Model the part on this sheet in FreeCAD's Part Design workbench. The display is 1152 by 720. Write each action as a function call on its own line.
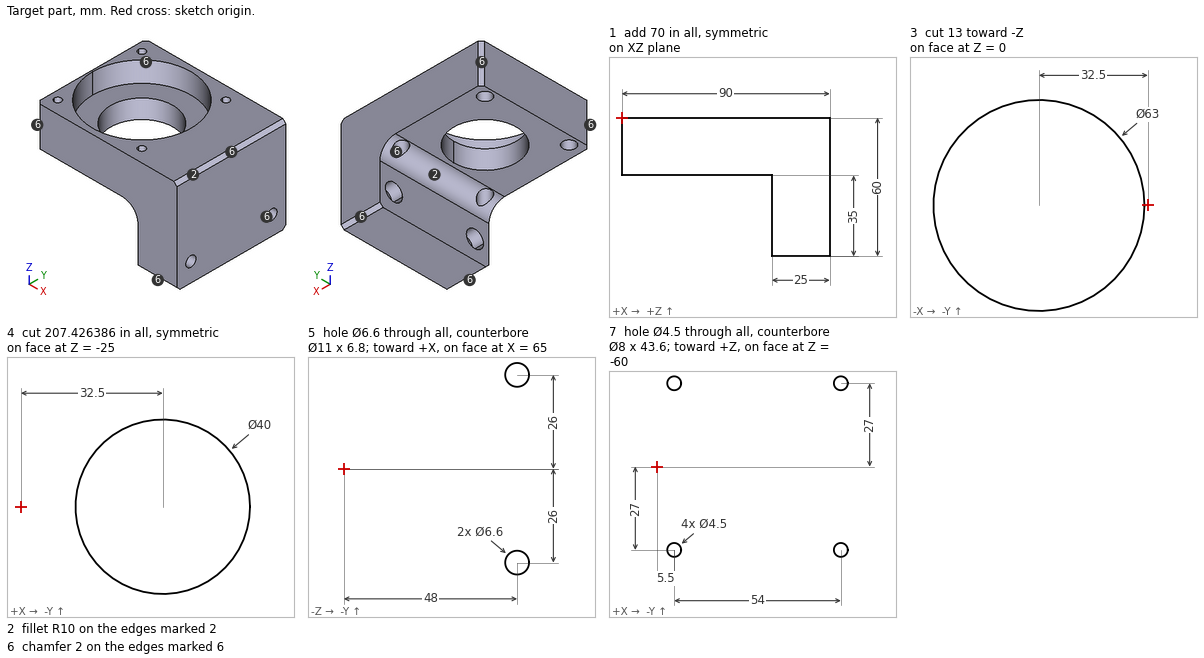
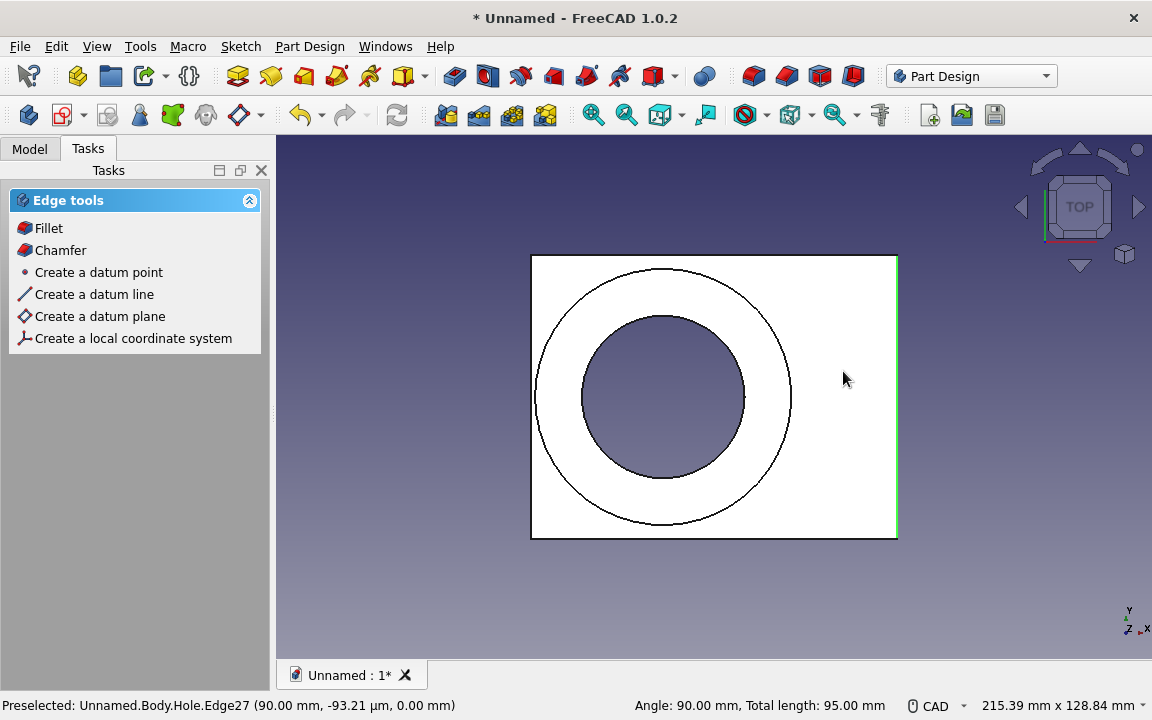
key(1)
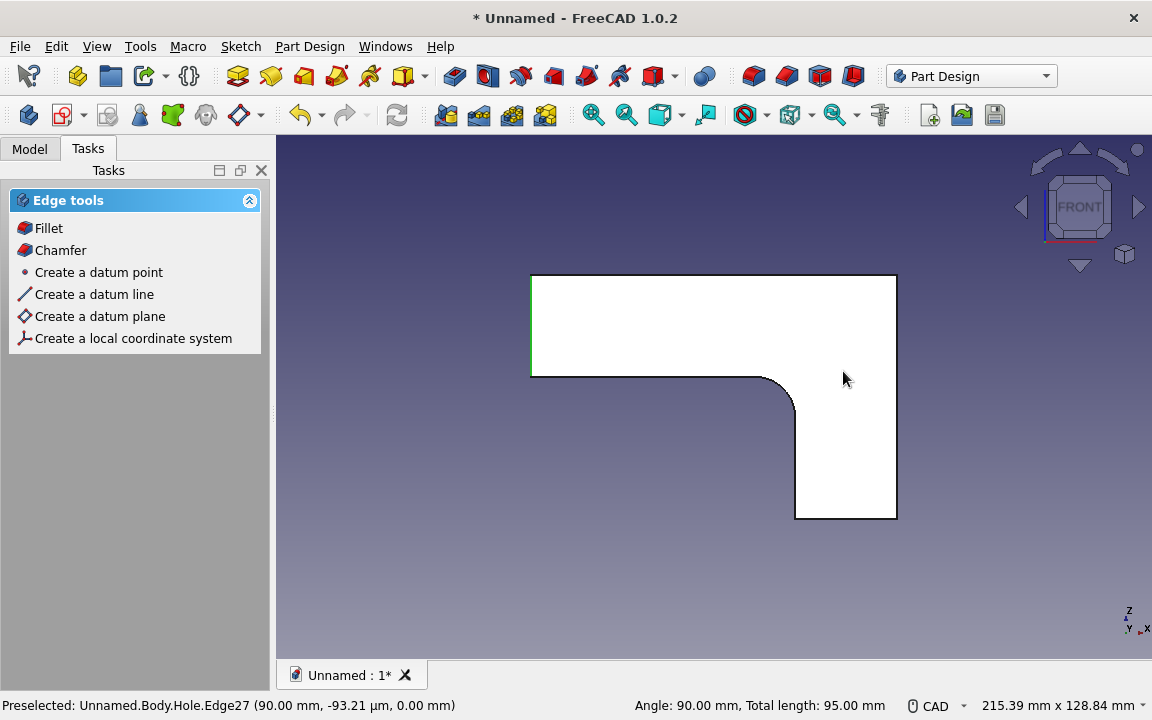
key(3)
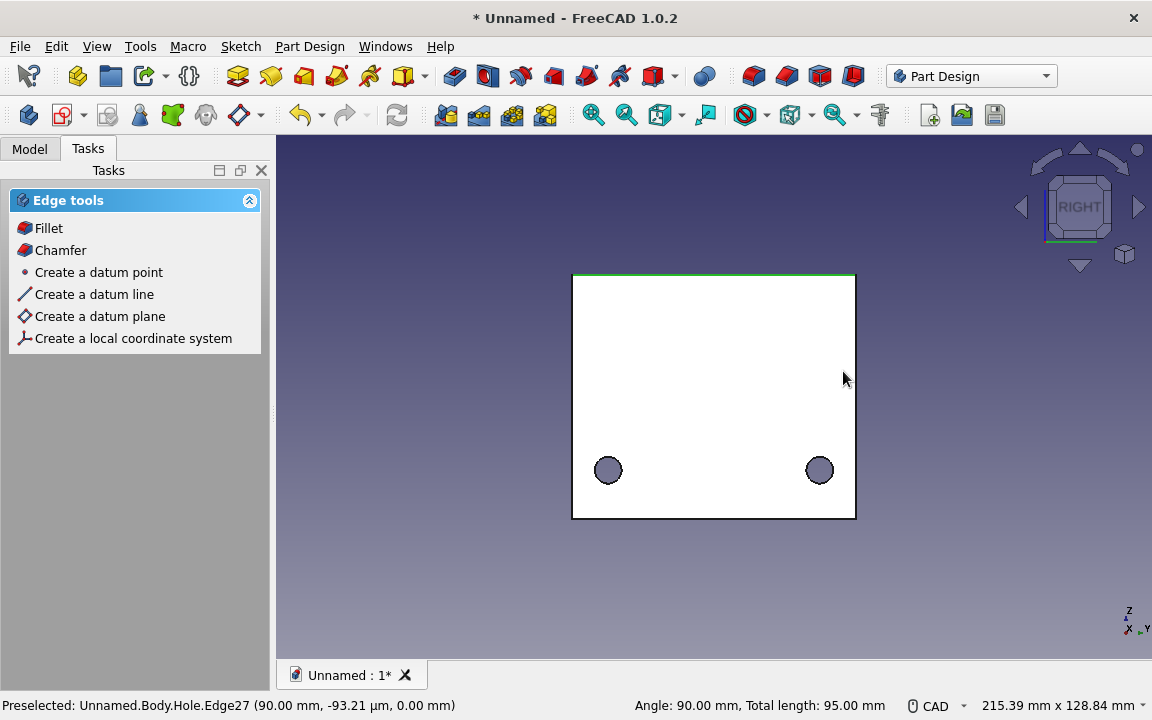
key(5)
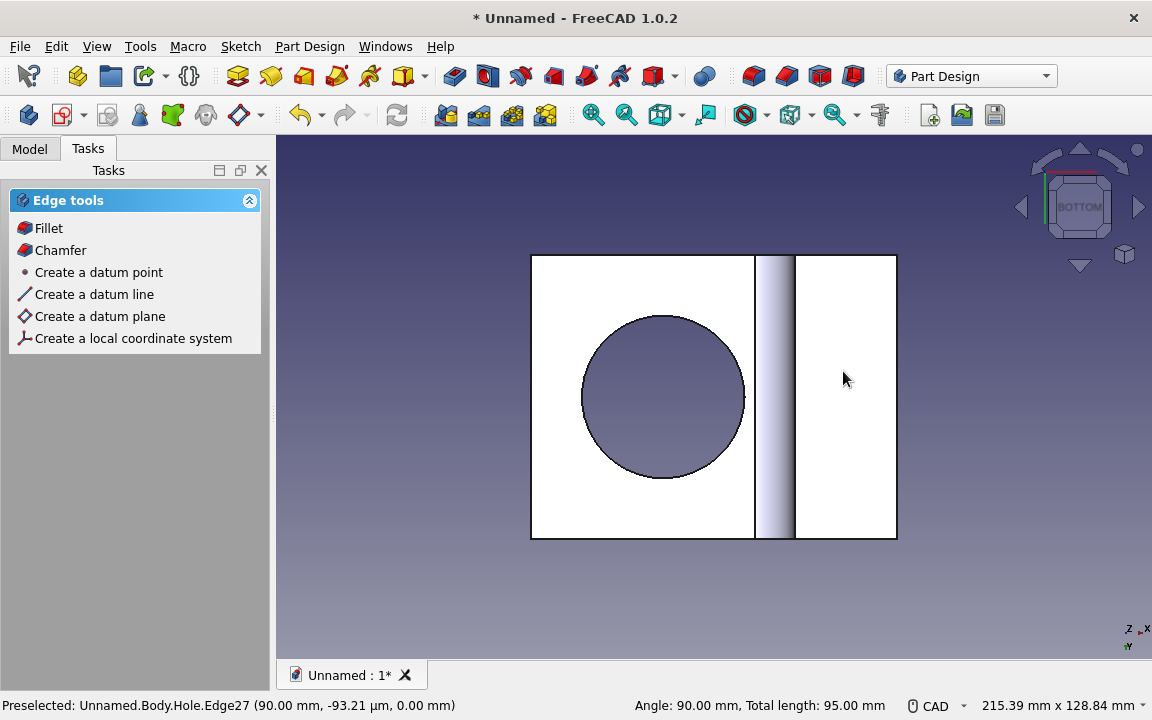
click(846, 254, ctrl)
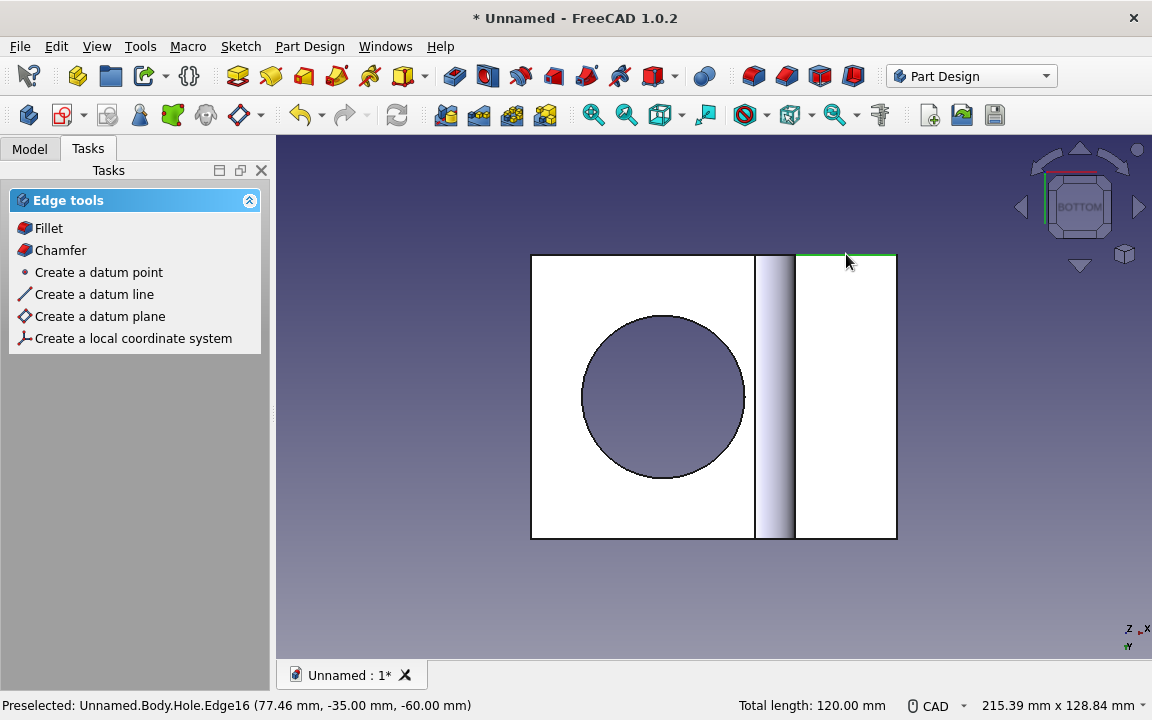
key(4)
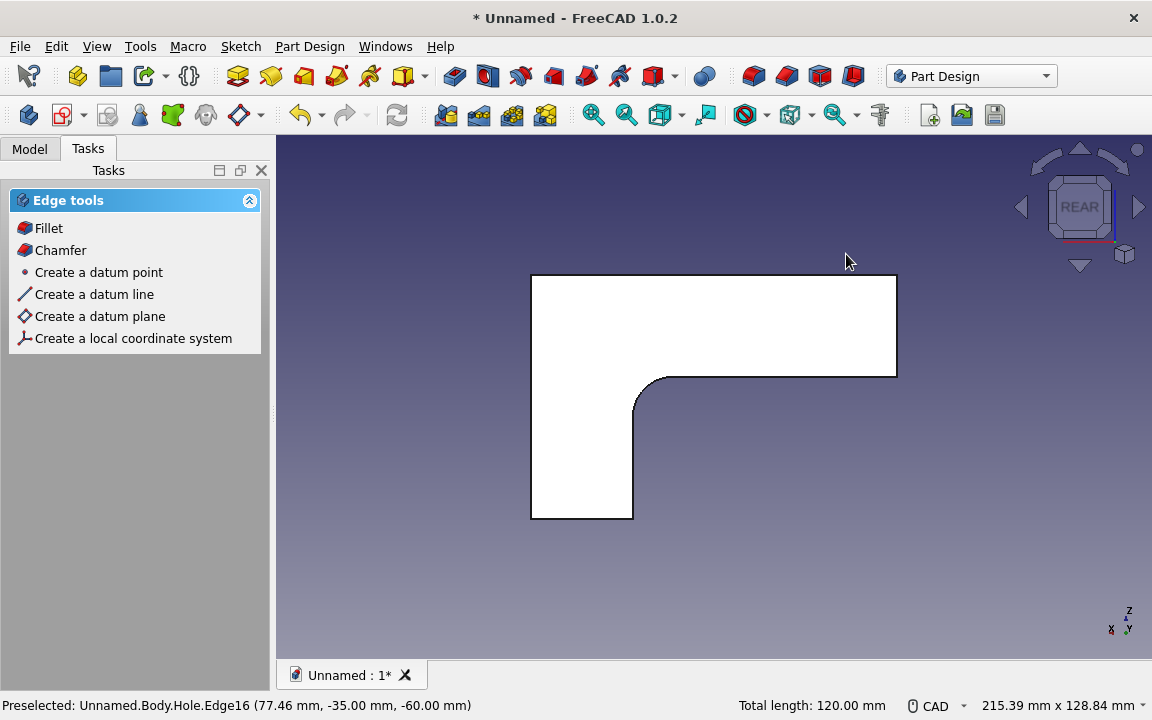
click(582, 518, ctrl)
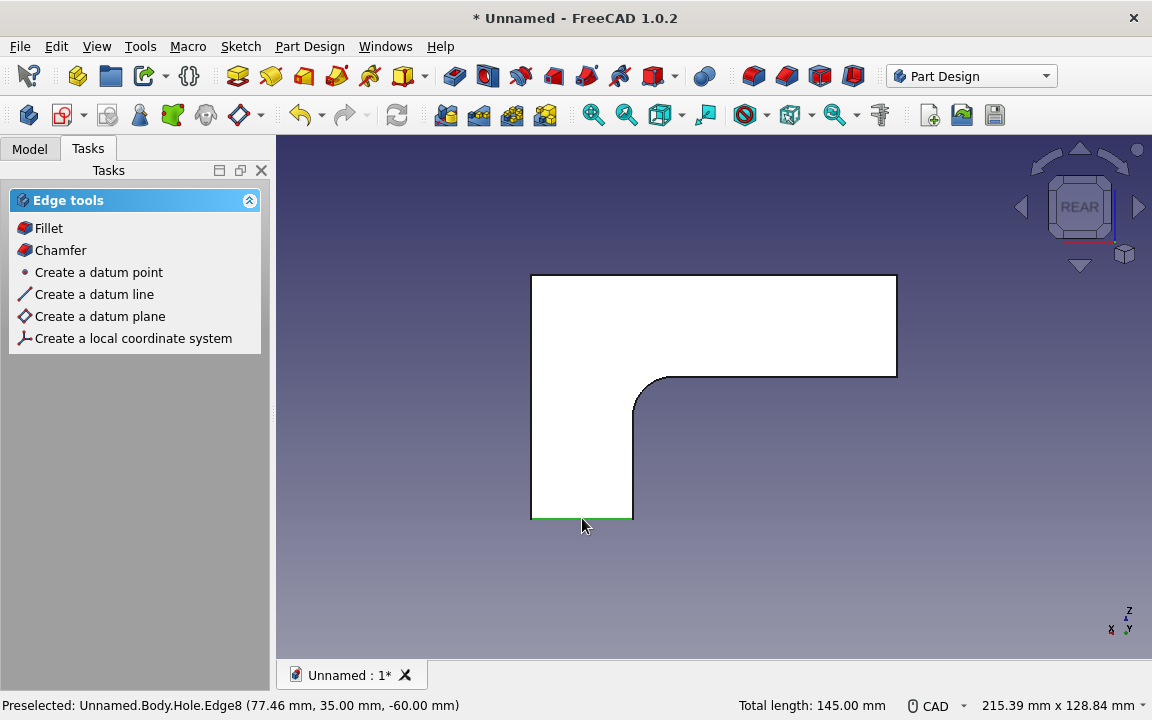
click(897, 325, ctrl)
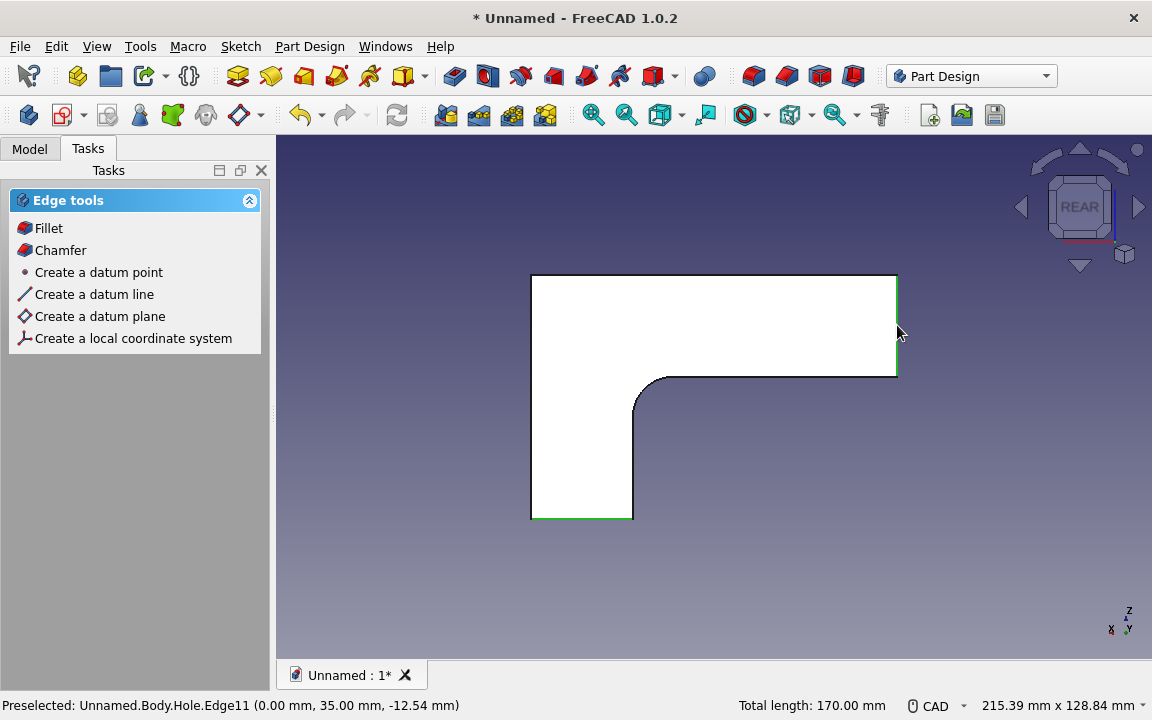
click(787, 76)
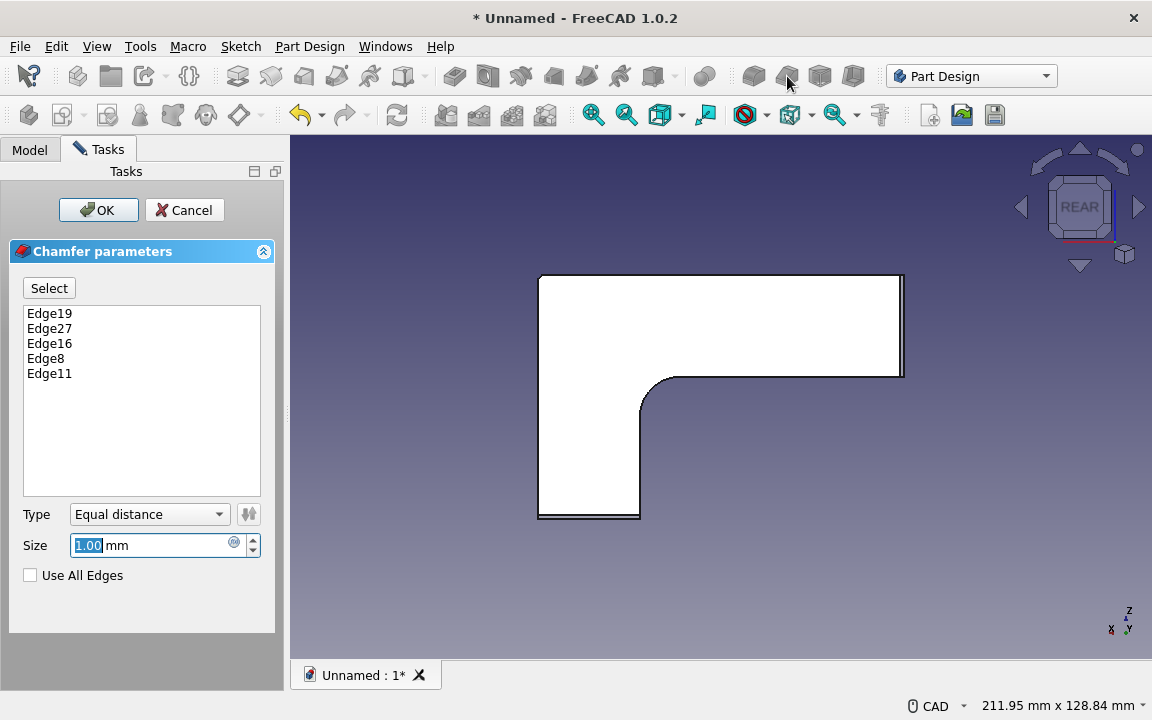
text(2)
key(Tab)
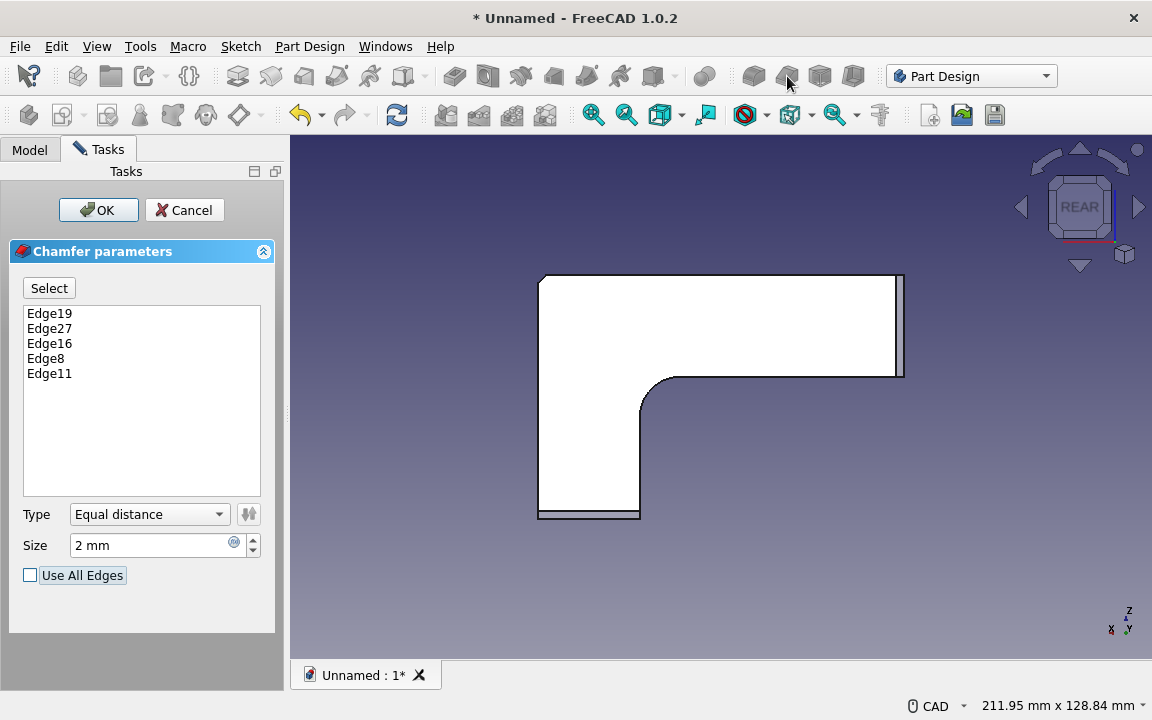
click(99, 210)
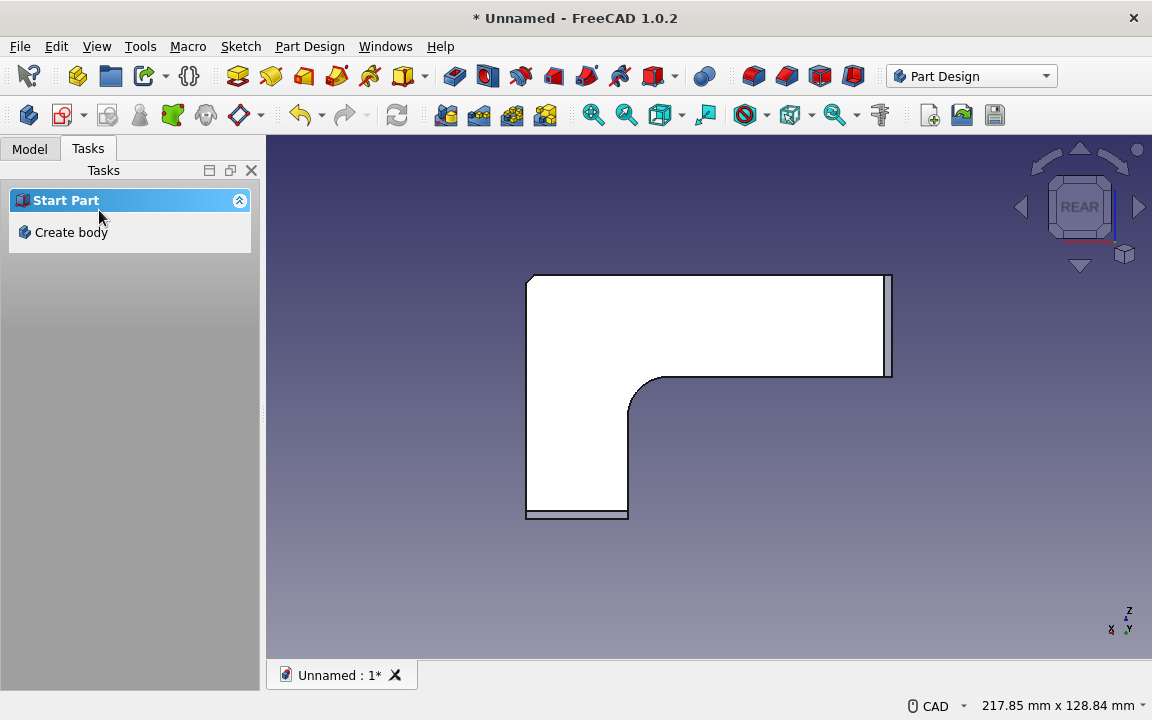
key(5)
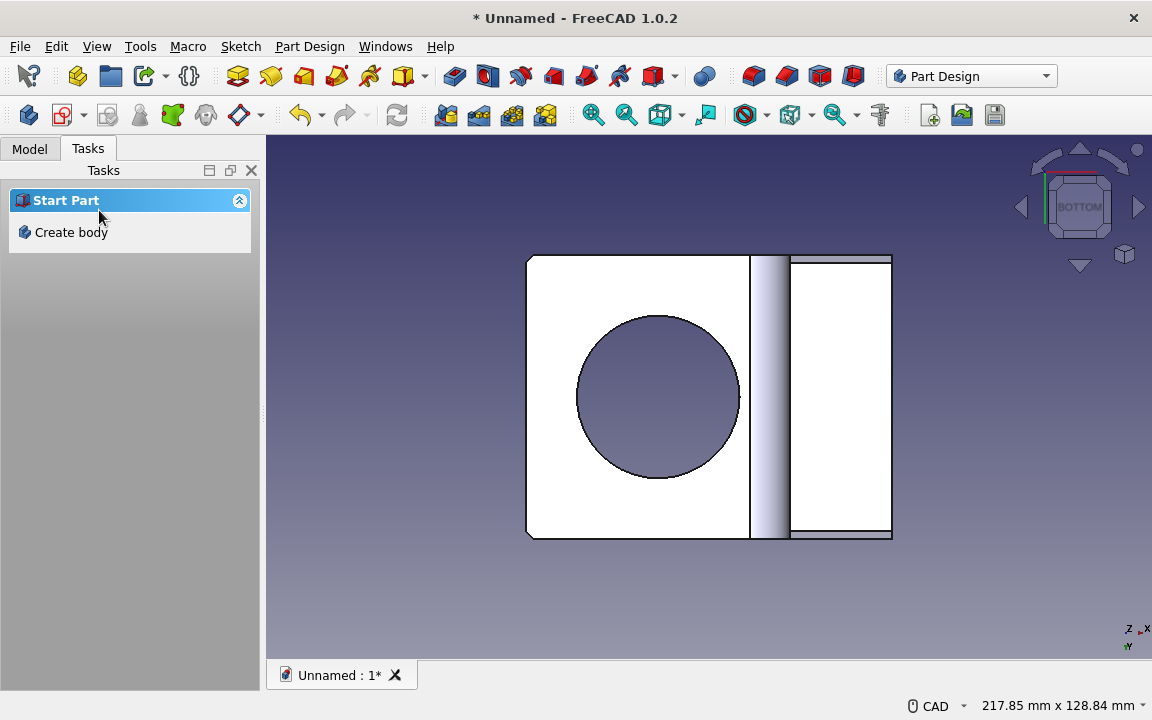
click(841, 473)